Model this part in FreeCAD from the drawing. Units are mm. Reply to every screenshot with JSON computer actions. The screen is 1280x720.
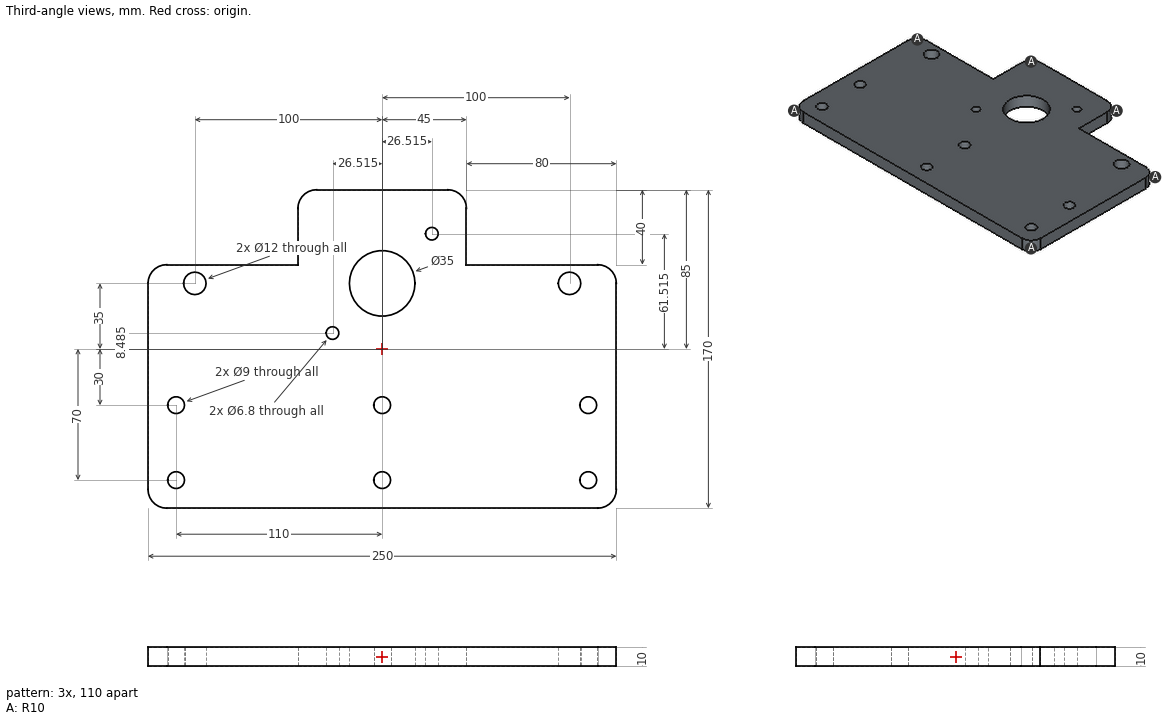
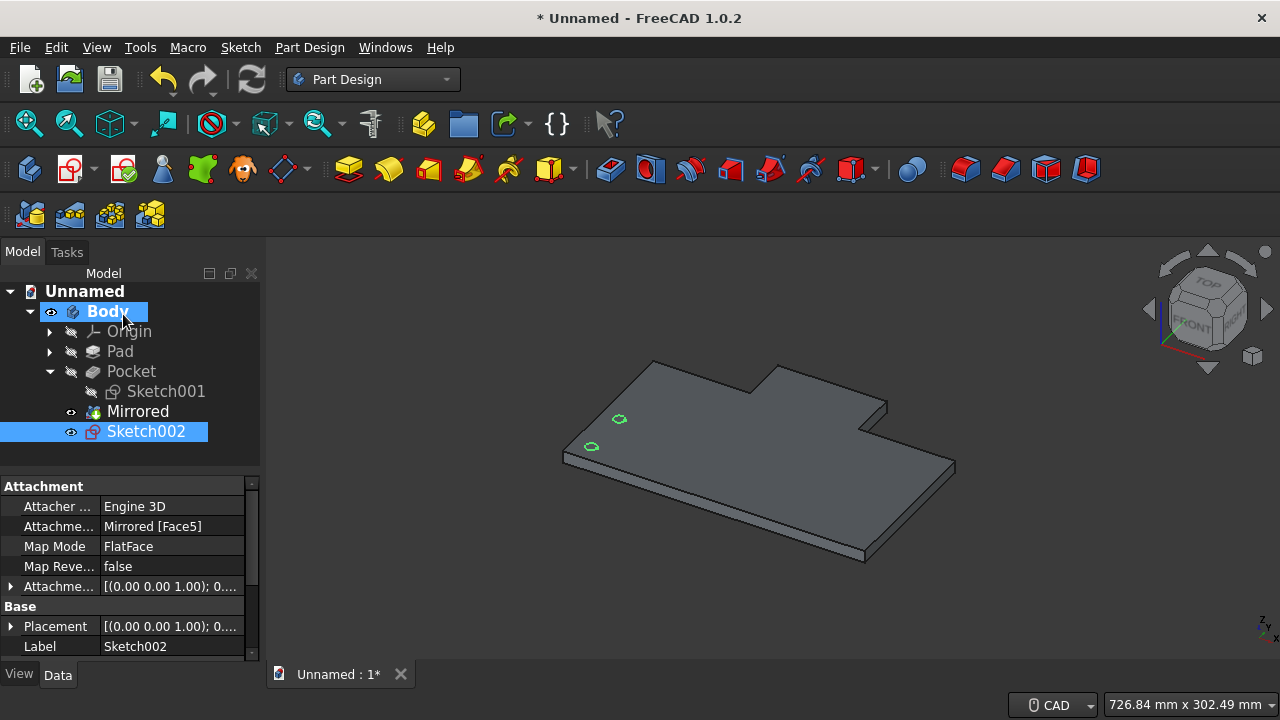
{"action": "left_click", "coordinate": [652, 170]}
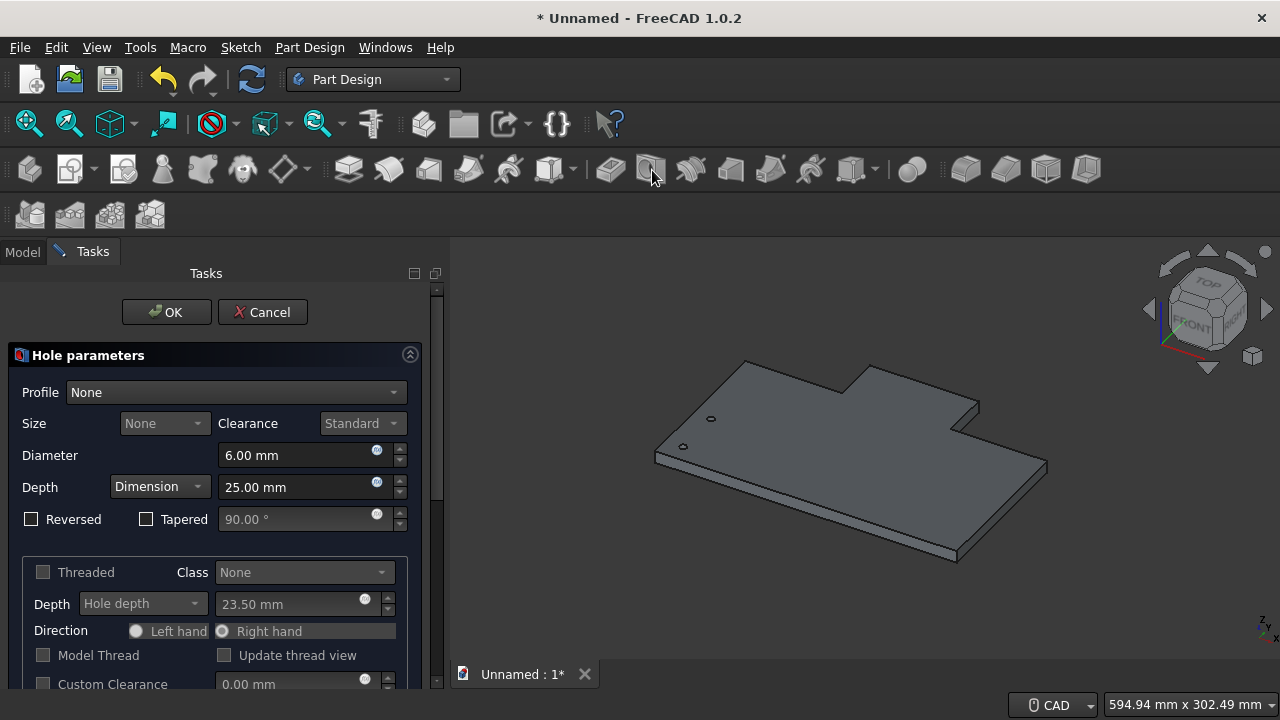
{"action": "triple_click", "coordinate": [305, 455]}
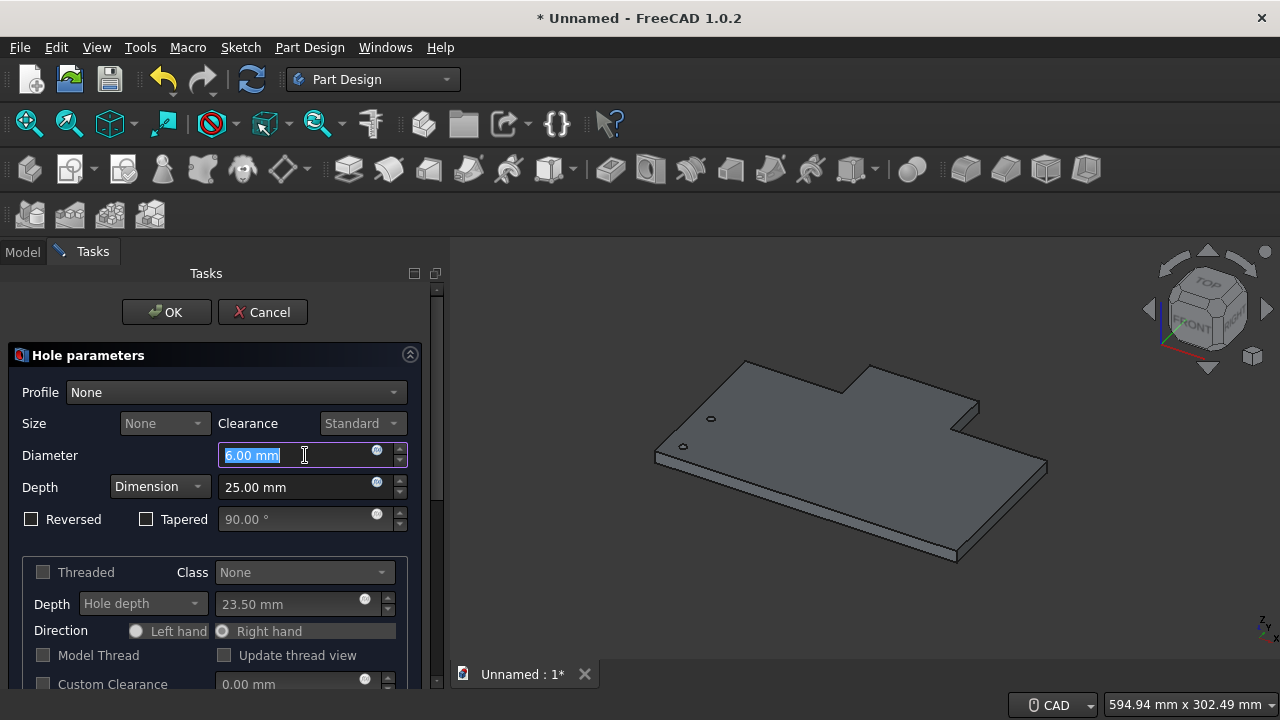
{"action": "type", "text": "9"}
{"action": "key", "text": "Tab"}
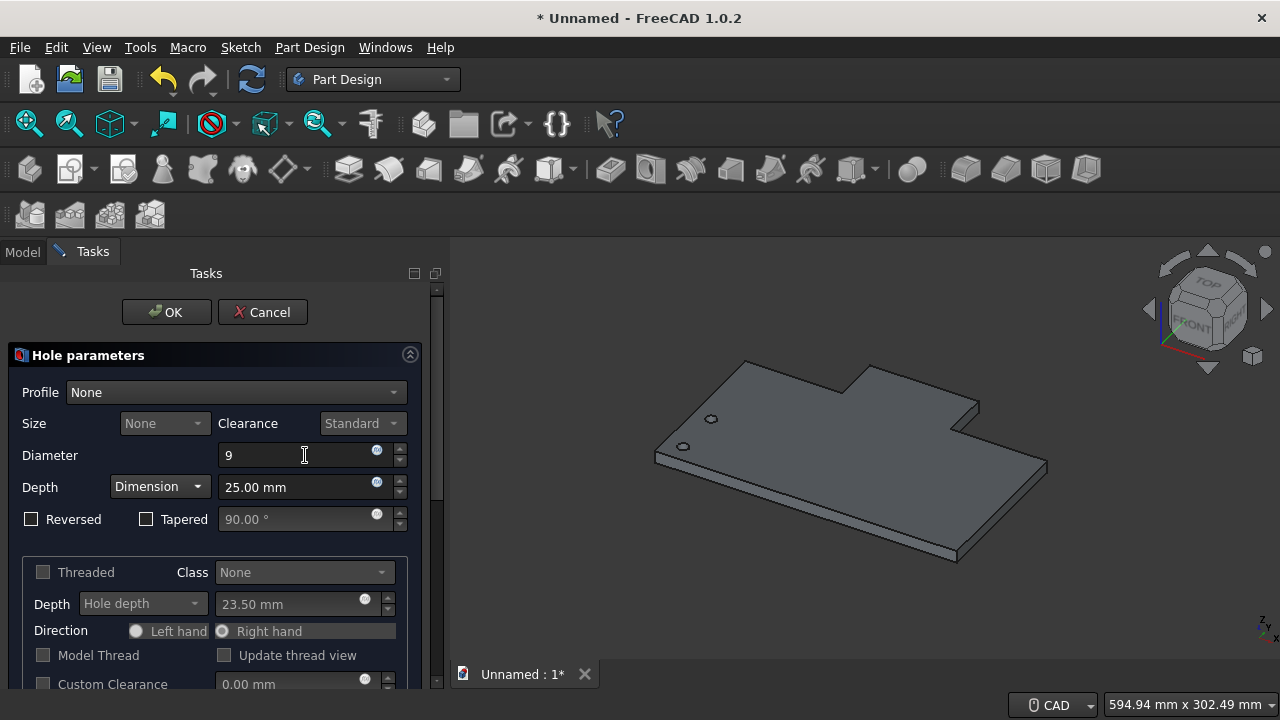
{"action": "left_click", "coordinate": [161, 486]}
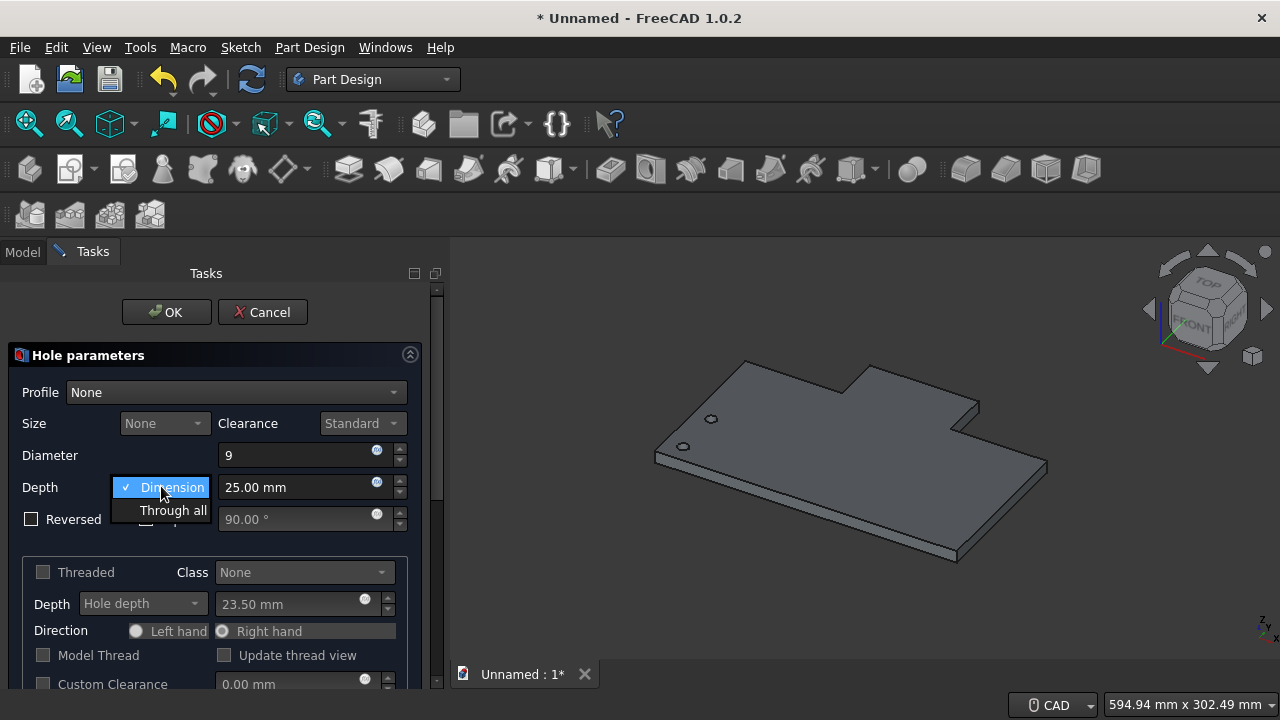
{"action": "left_click", "coordinate": [160, 510]}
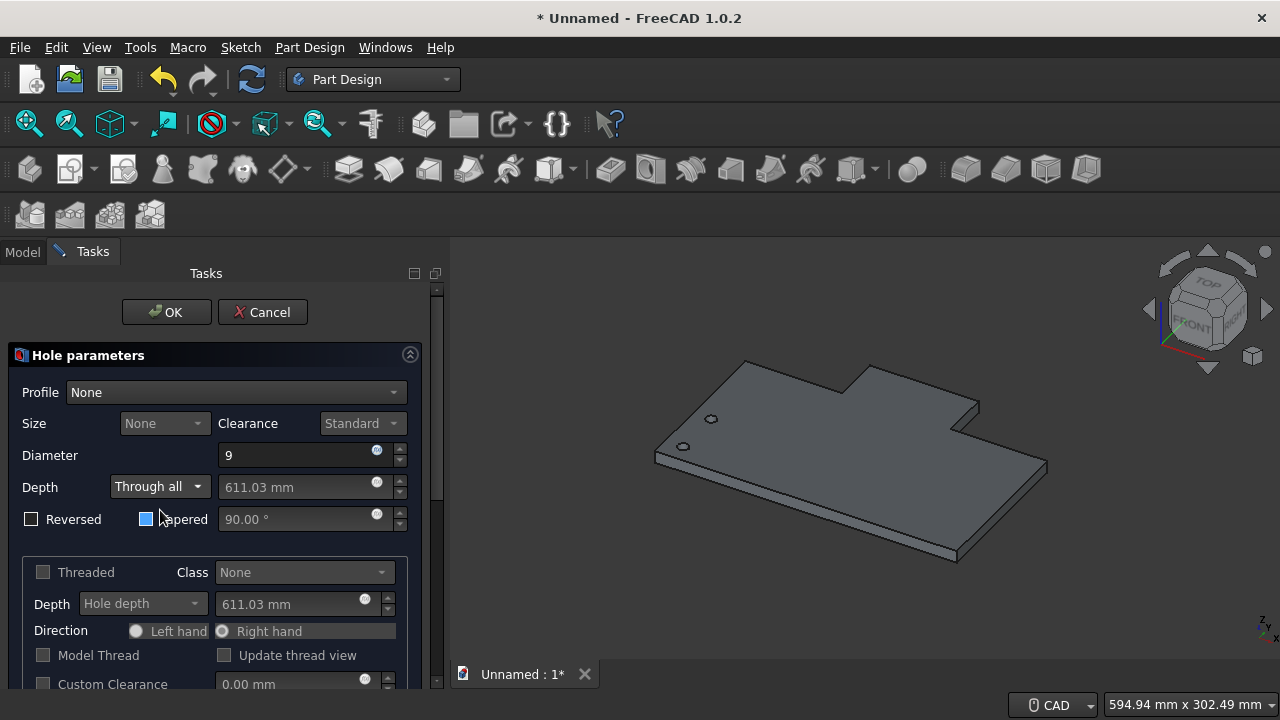
{"action": "left_click", "coordinate": [167, 312]}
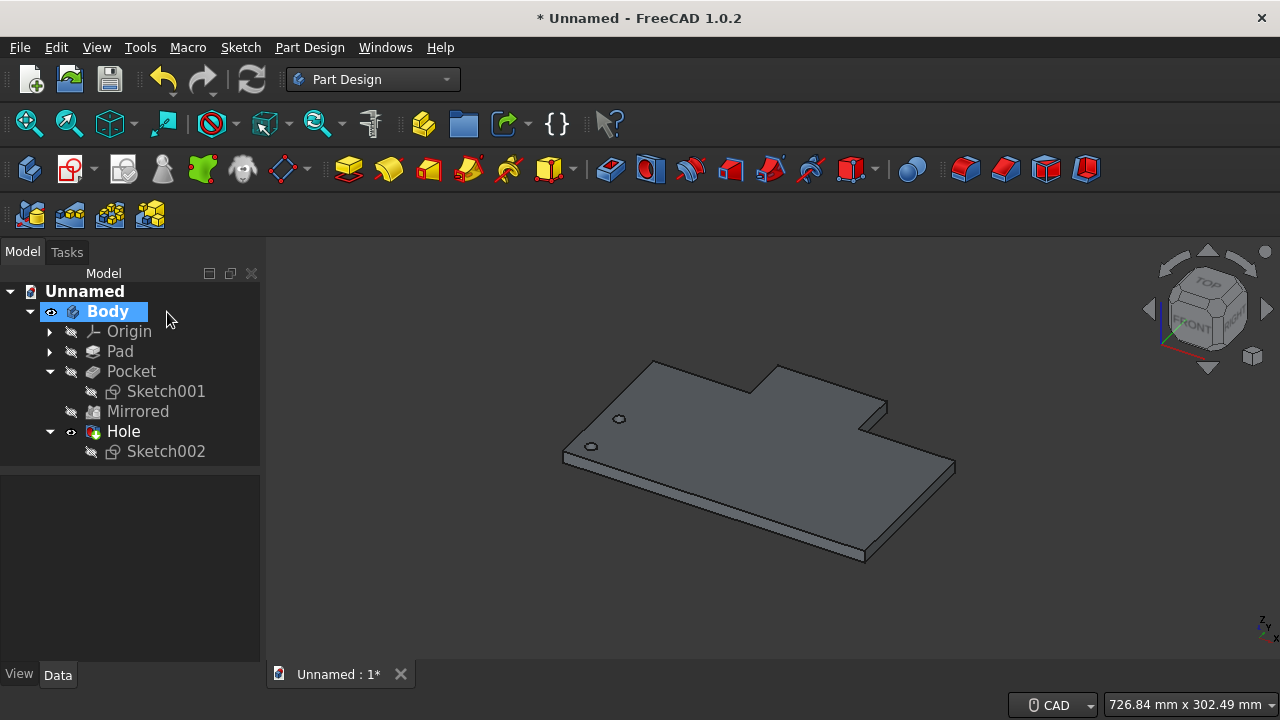
{"action": "left_click", "coordinate": [116, 432]}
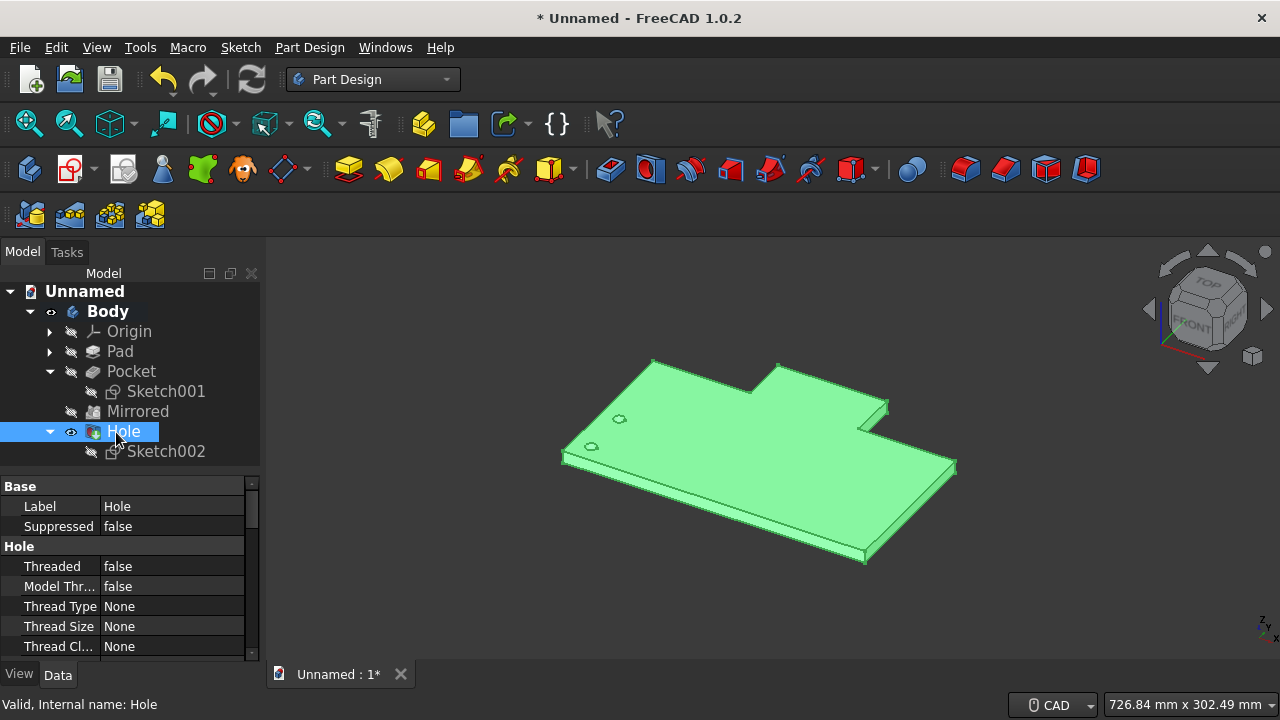
{"action": "left_click", "coordinate": [70, 214]}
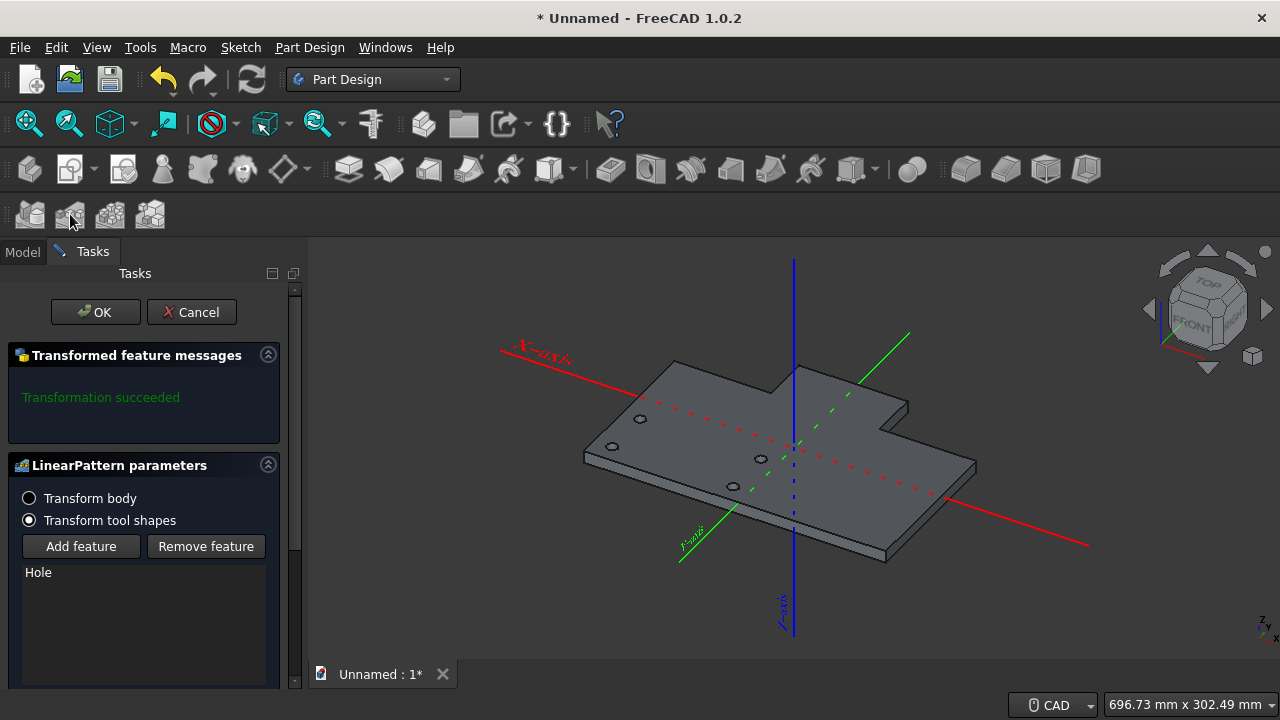
{"action": "scroll", "coordinate": [295, 486], "scroll_direction": "down", "scroll_amount": 2}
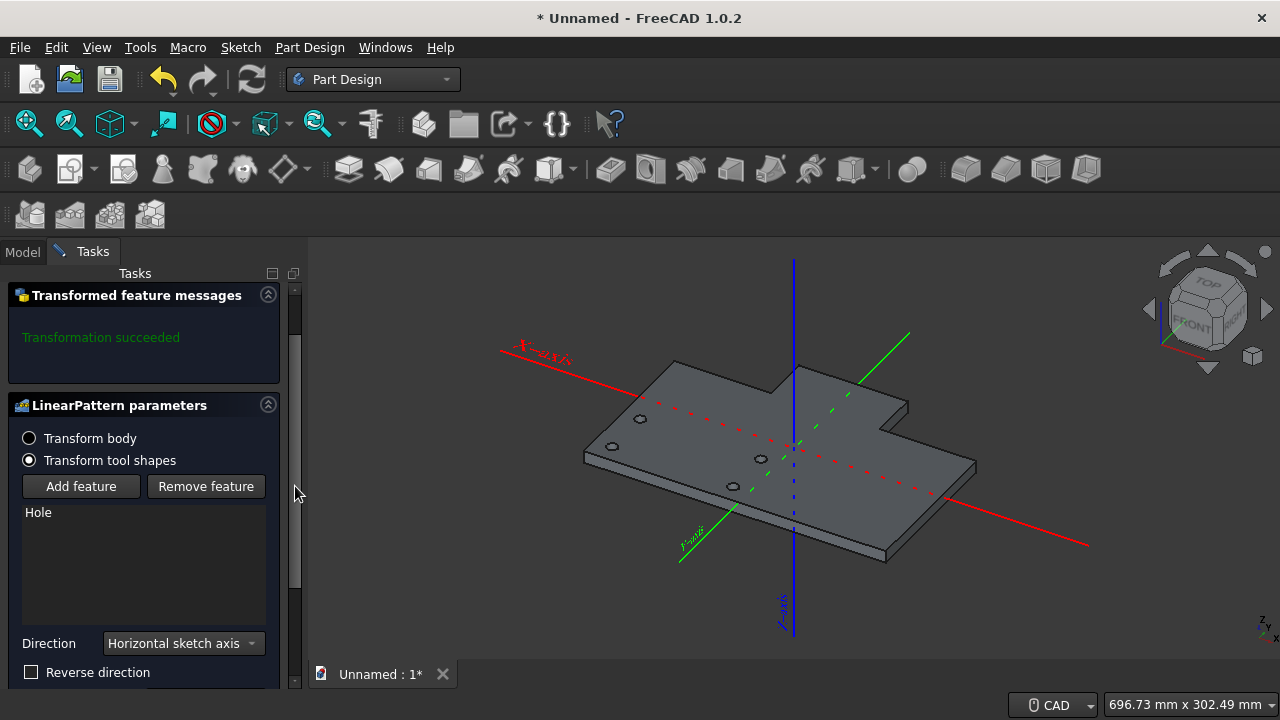
{"action": "left_click", "coordinate": [184, 584]}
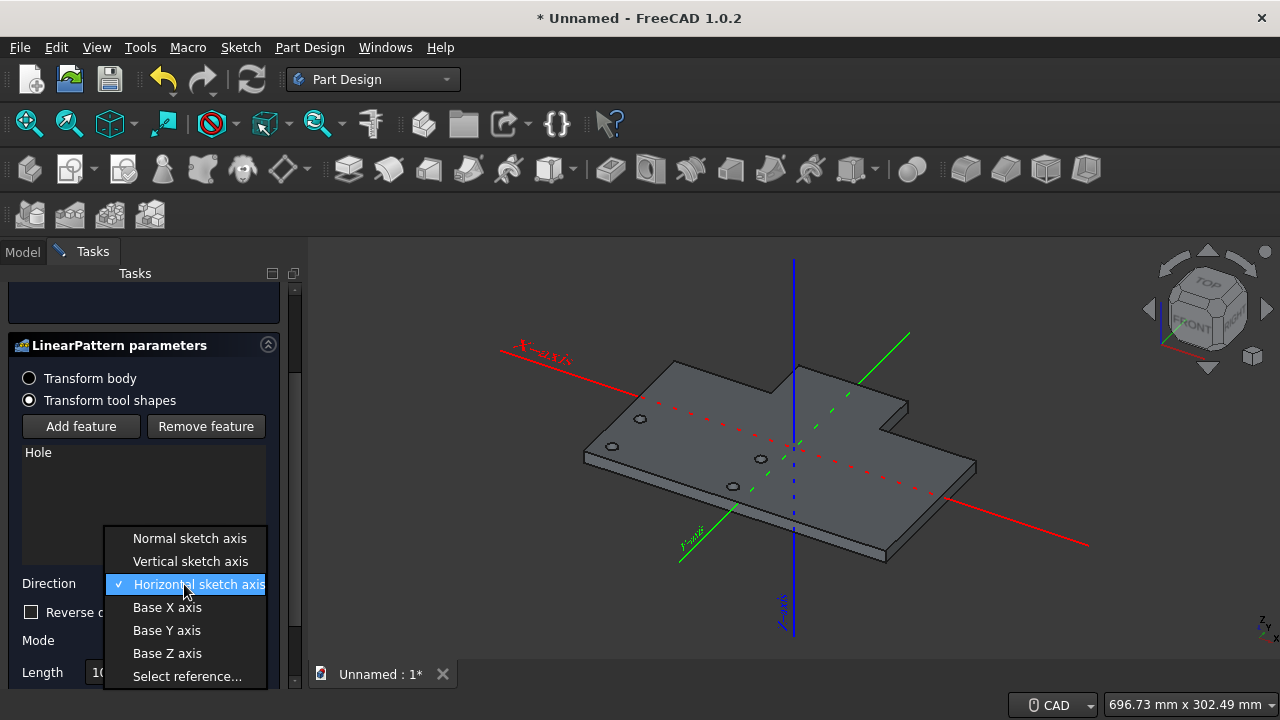
{"action": "left_click", "coordinate": [184, 608]}